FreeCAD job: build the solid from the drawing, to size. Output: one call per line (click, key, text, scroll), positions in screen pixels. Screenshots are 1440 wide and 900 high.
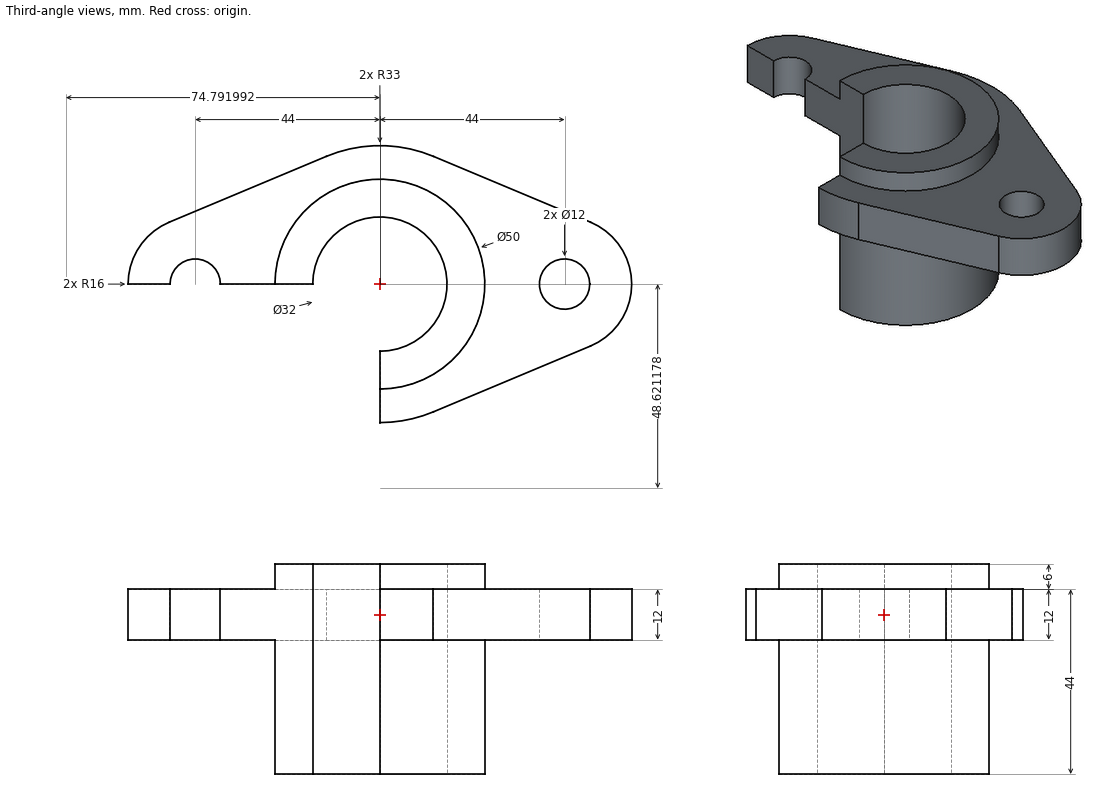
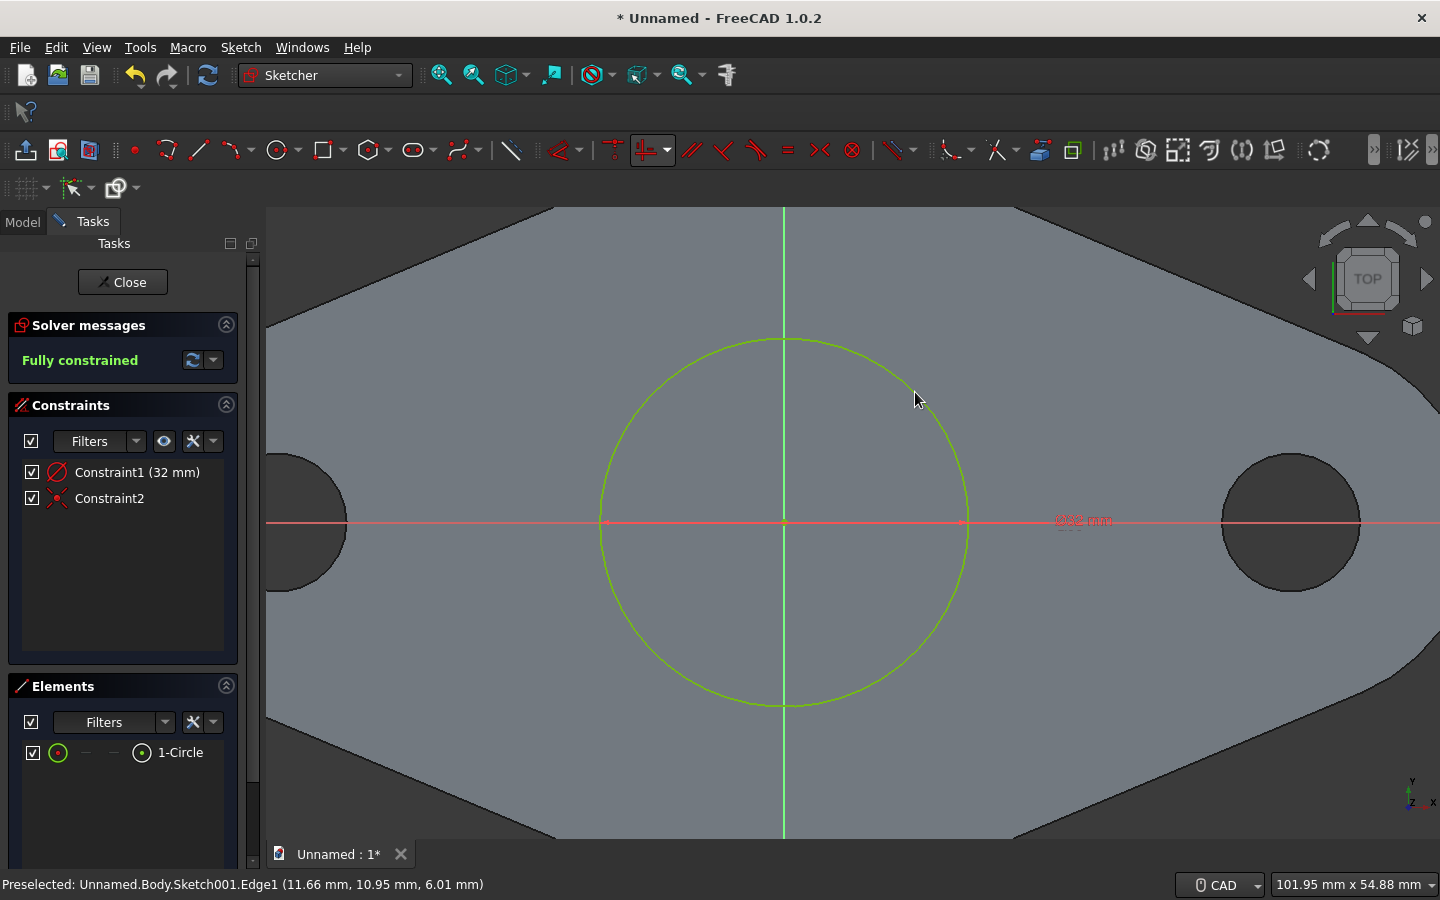
click(123, 282)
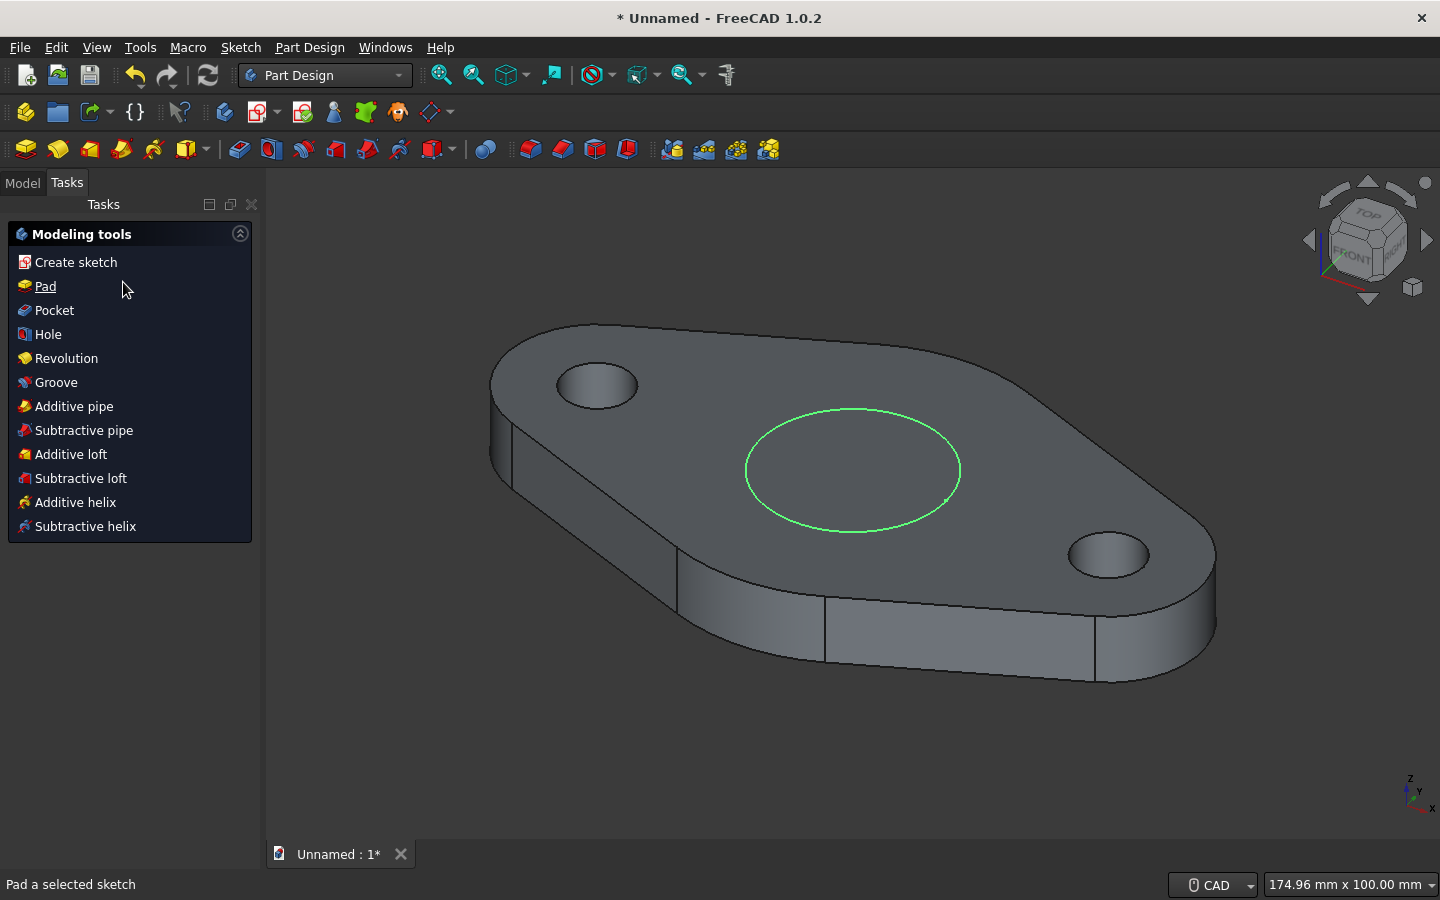
click(240, 150)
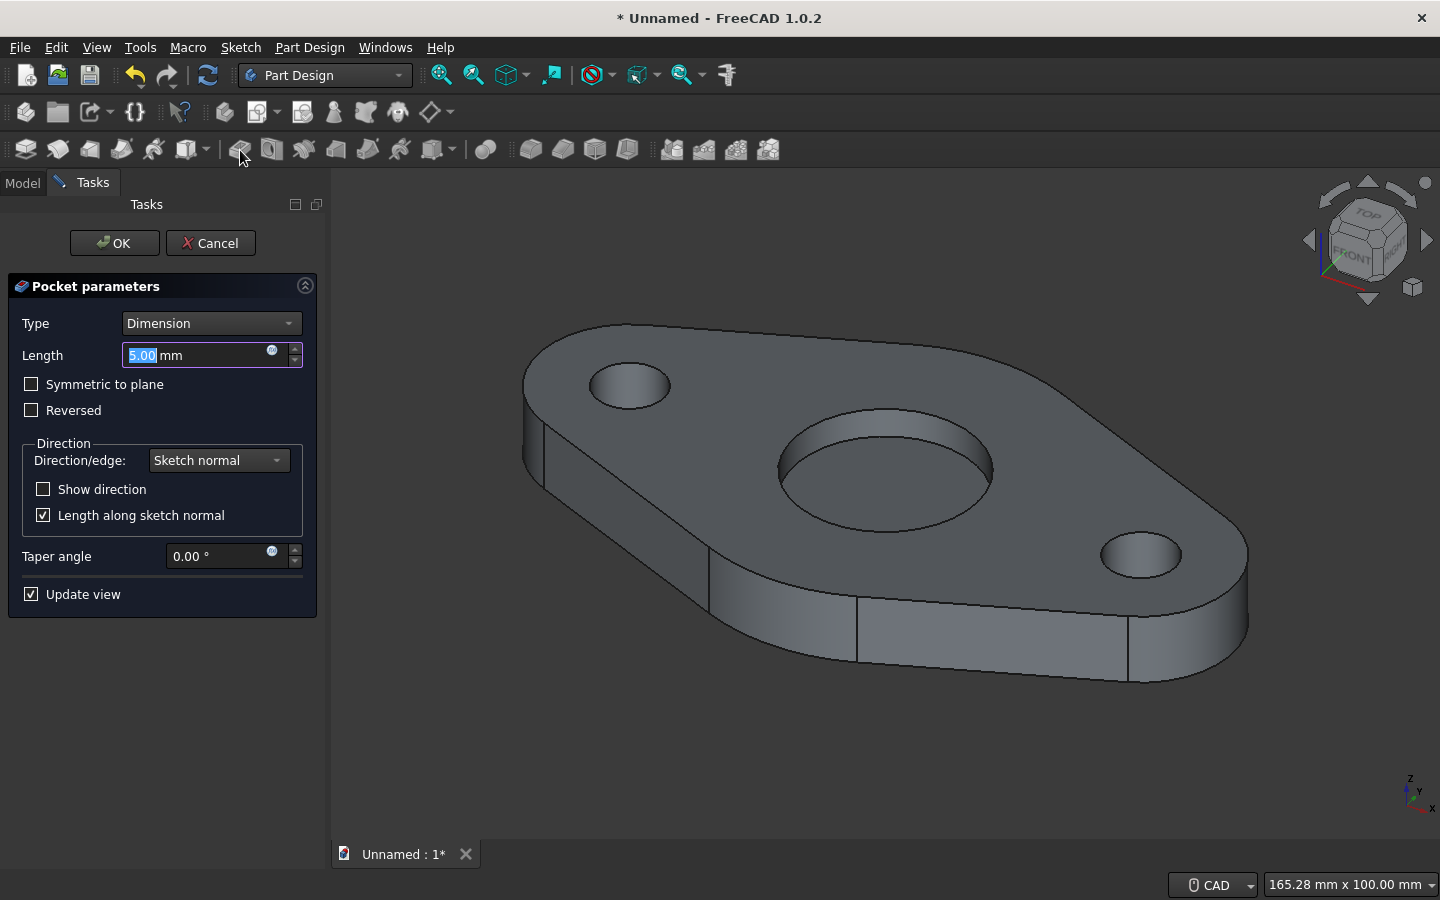
text(12)
key(Tab)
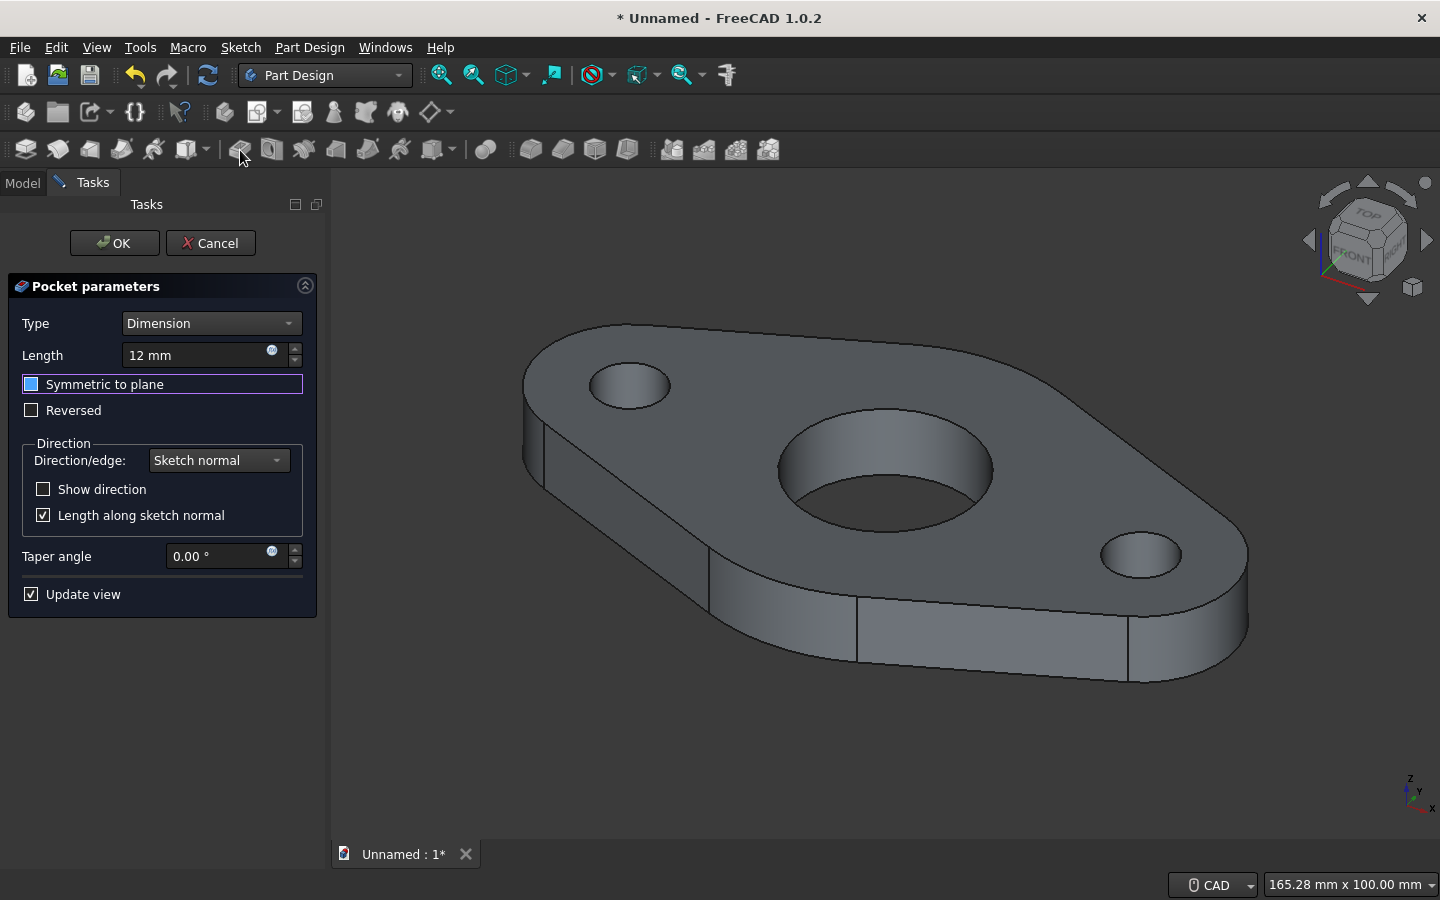
click(115, 243)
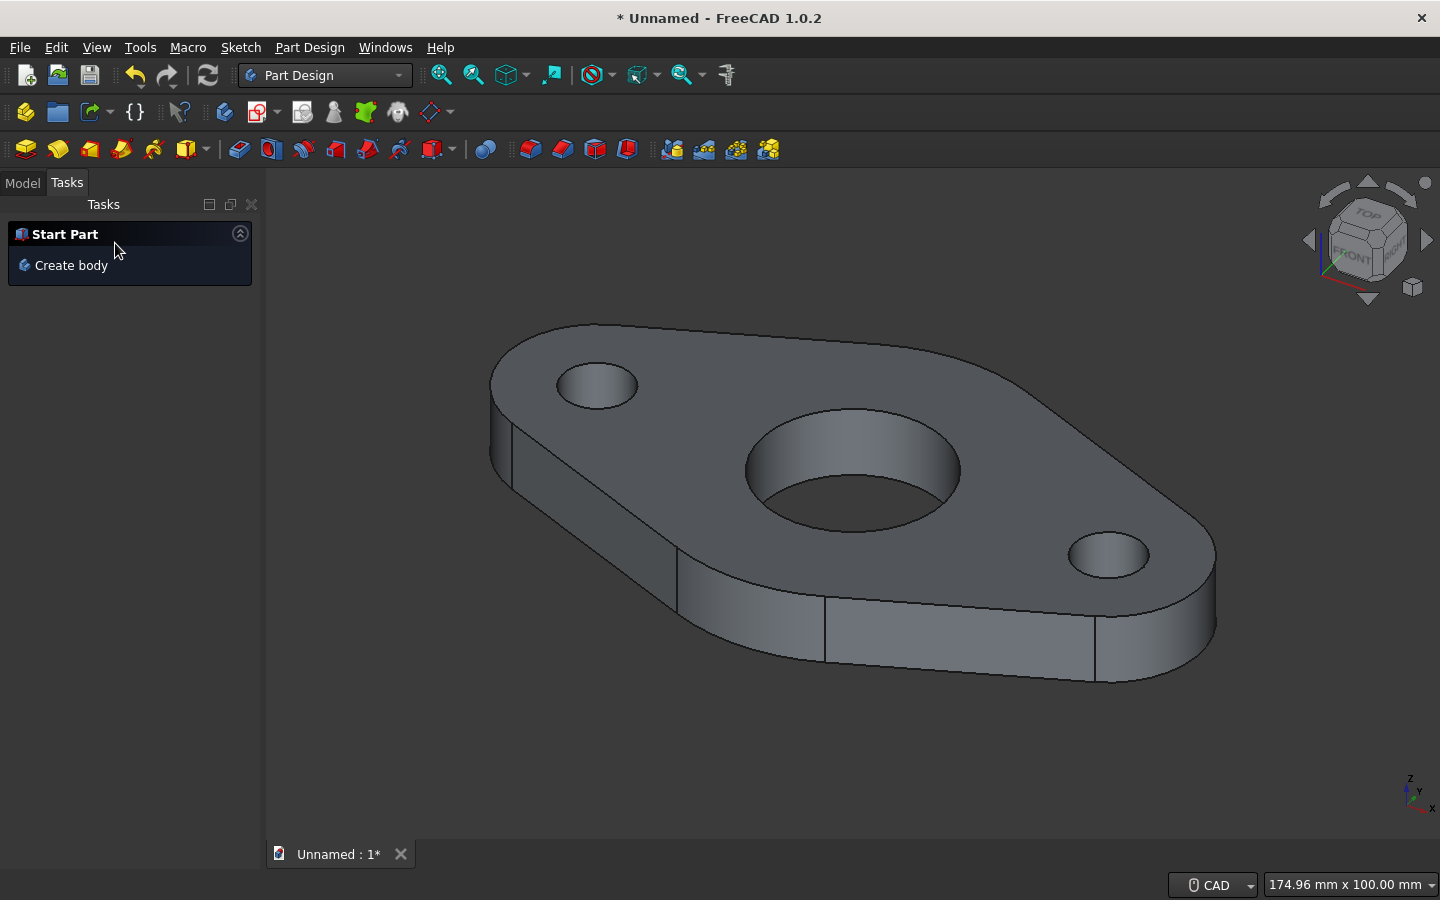
click(889, 565)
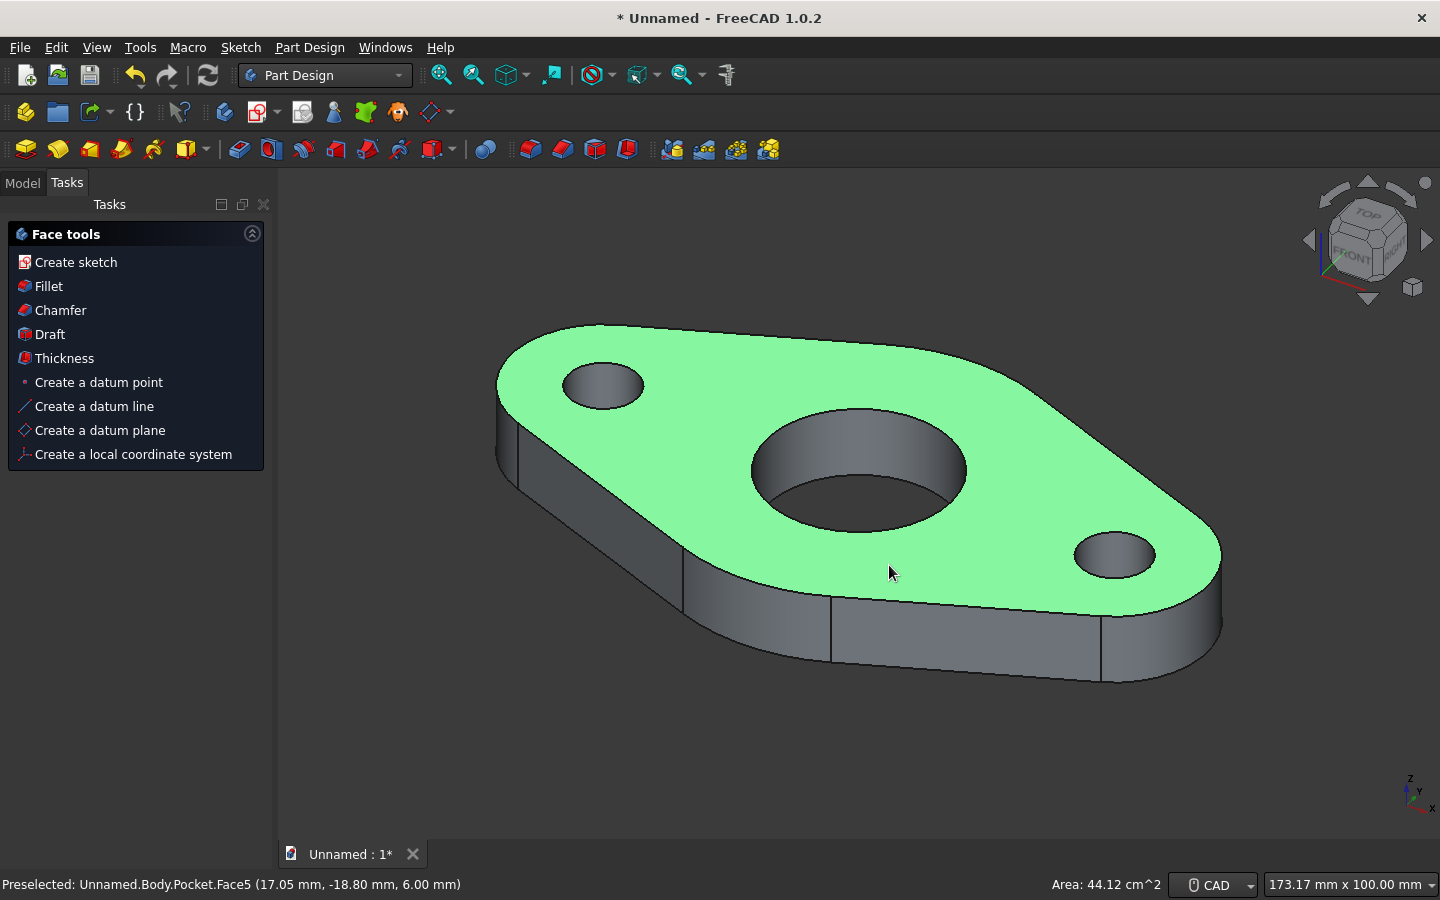
click(258, 112)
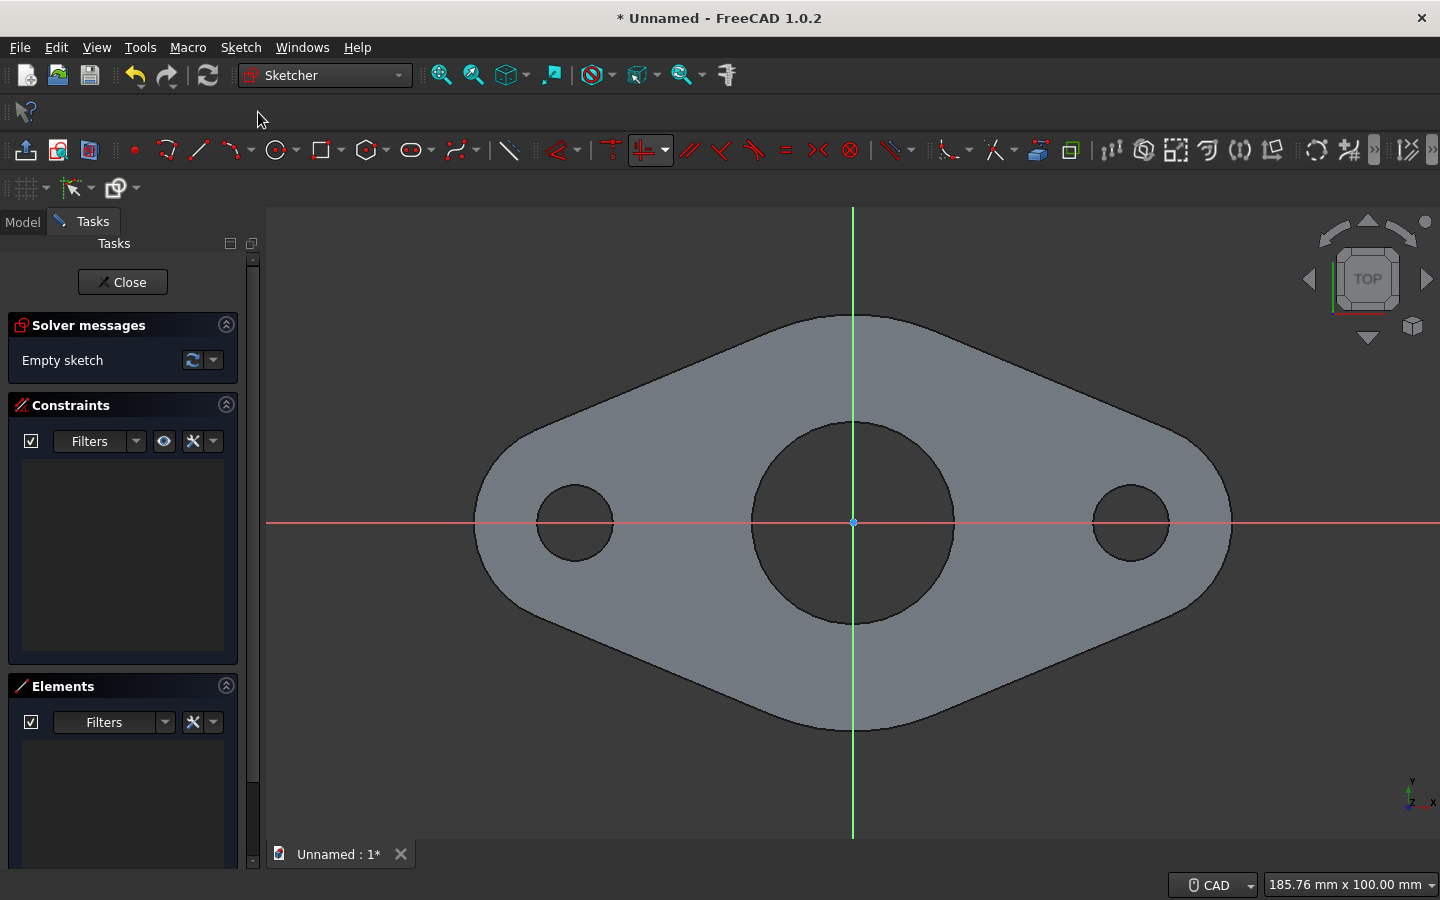
key(g)
key(c)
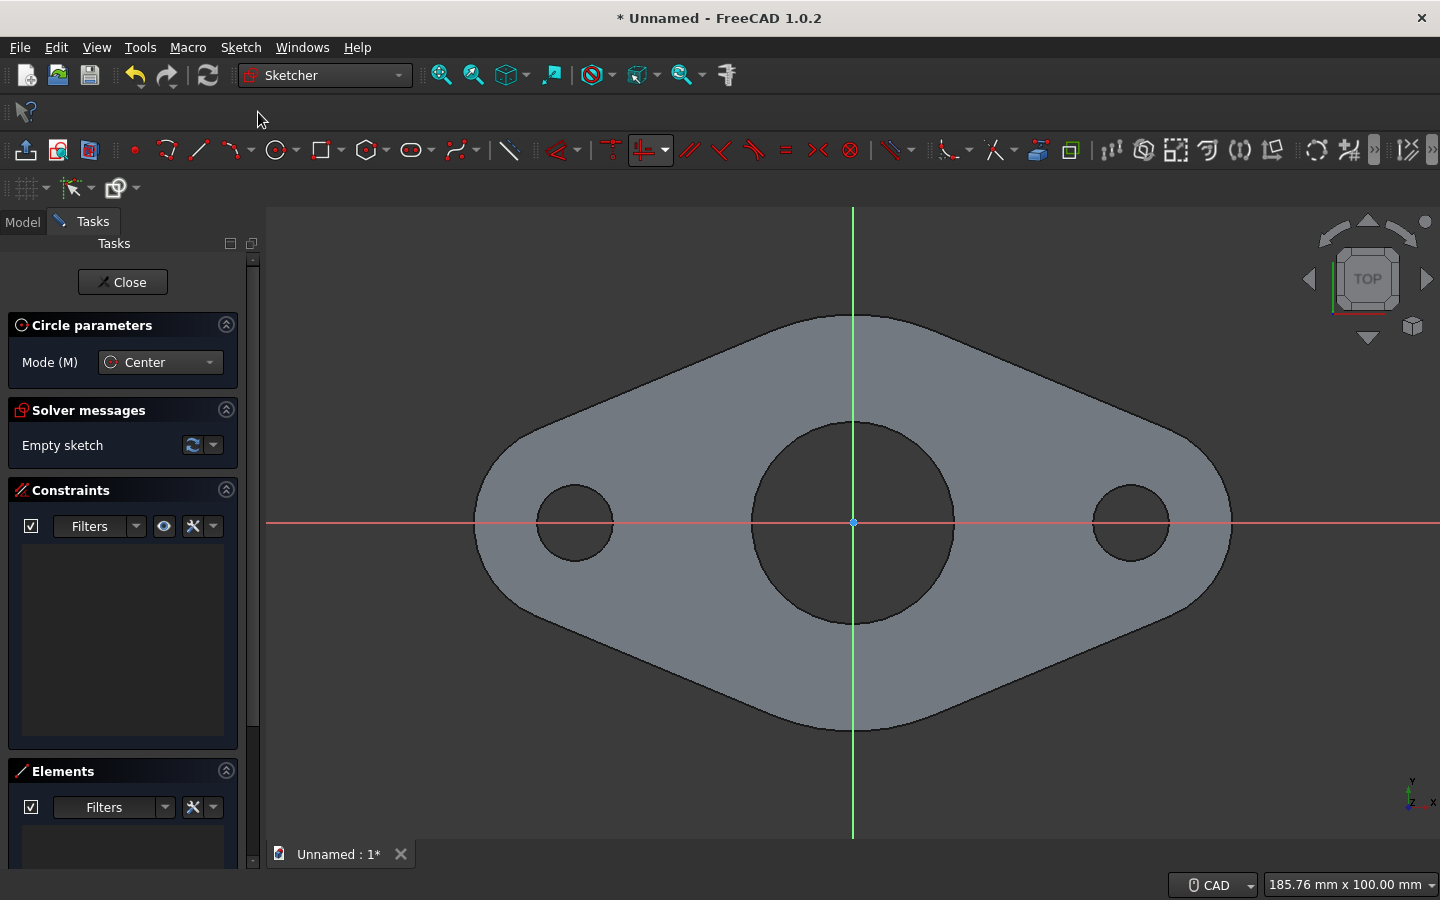
click(853, 523)
move(965, 411)